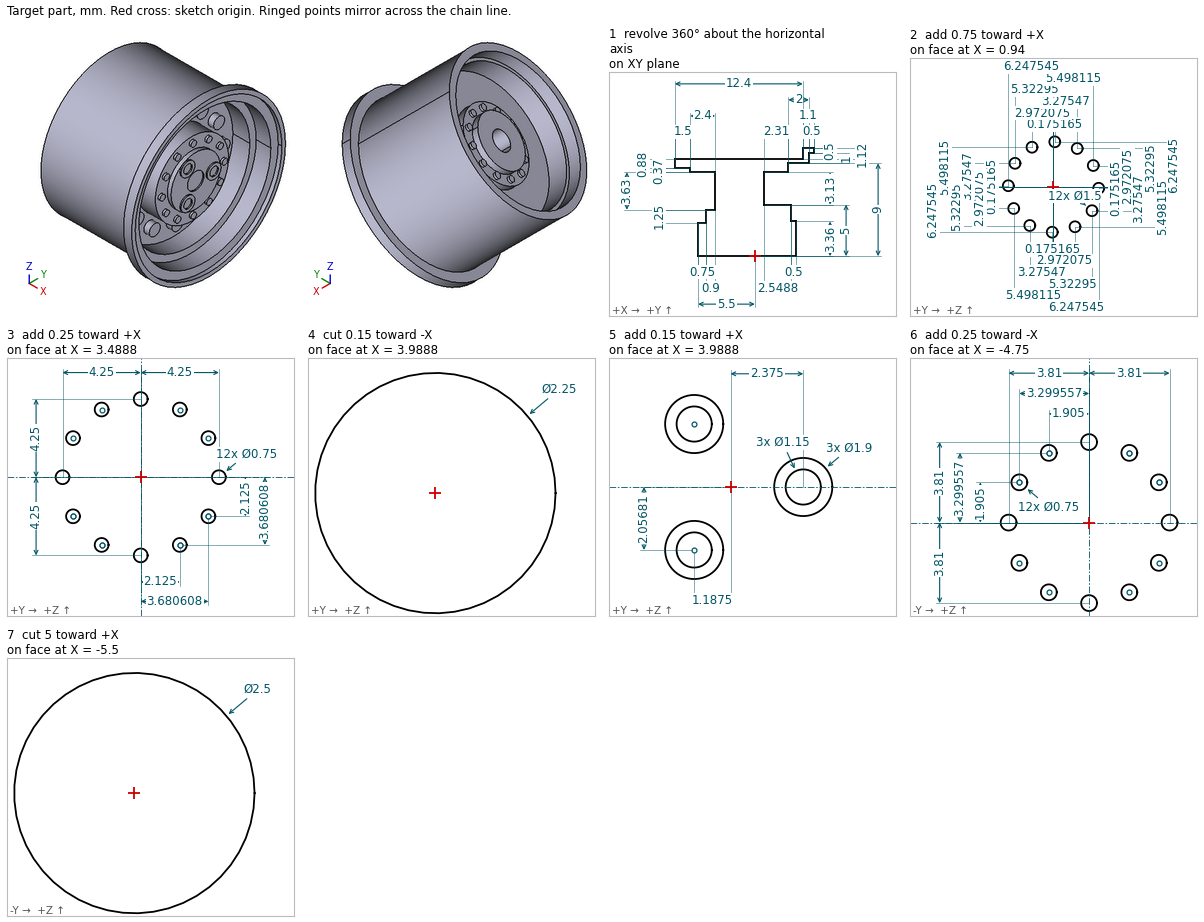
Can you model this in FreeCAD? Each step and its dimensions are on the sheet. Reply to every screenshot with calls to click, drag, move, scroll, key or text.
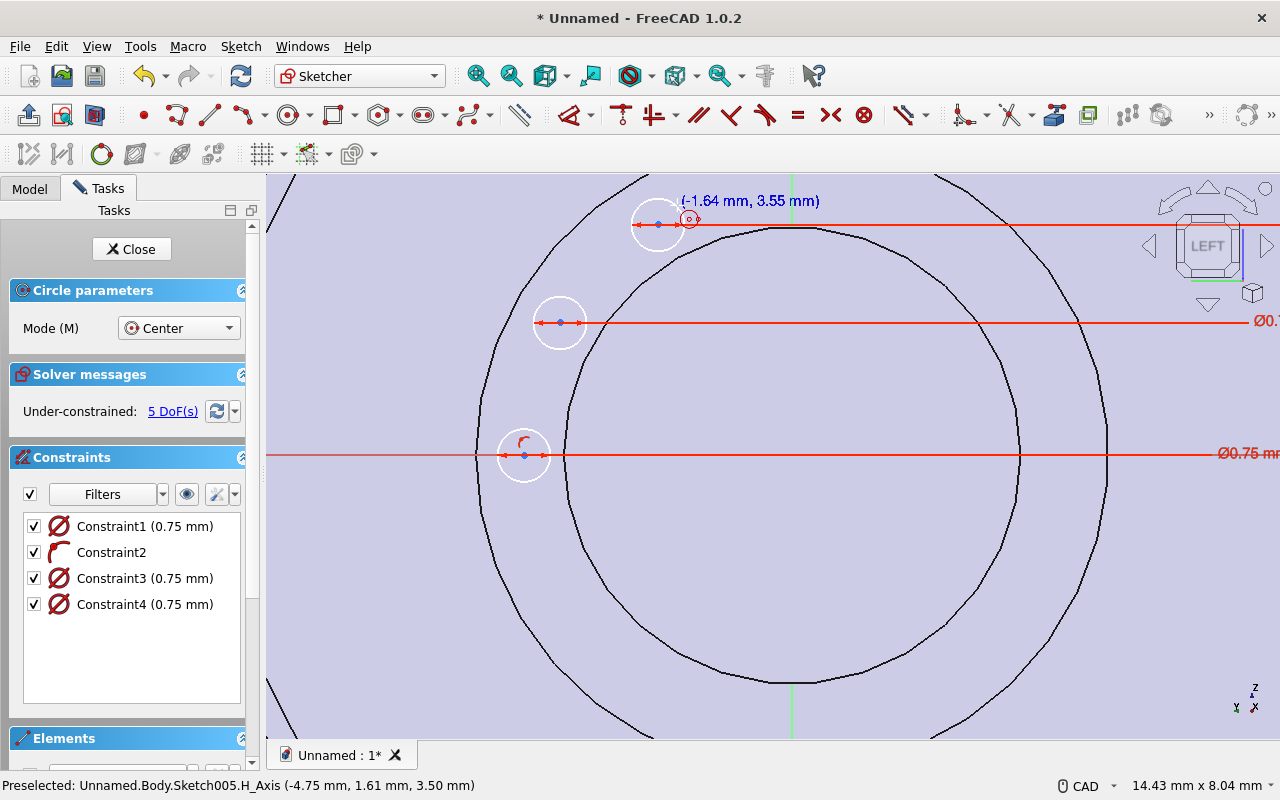
scroll(526, 459, down, 2)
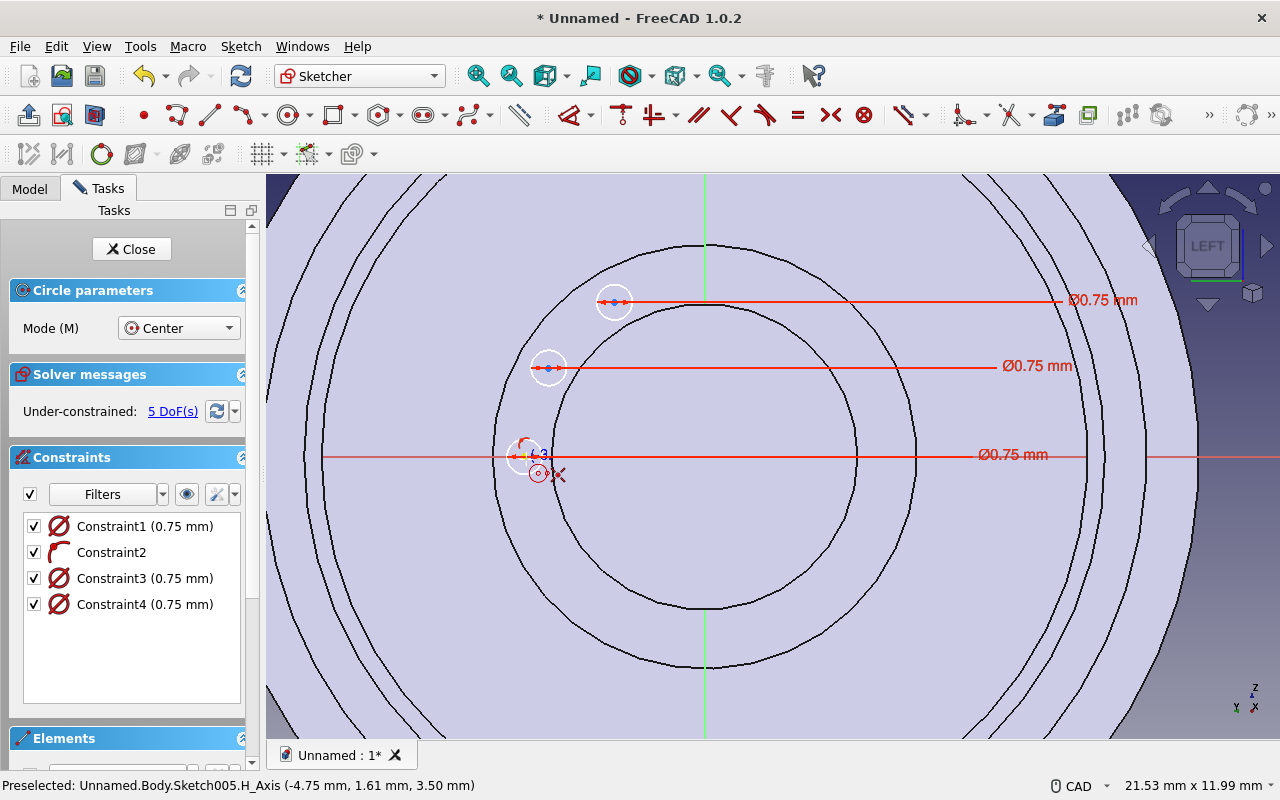
scroll(705, 277, up, 2)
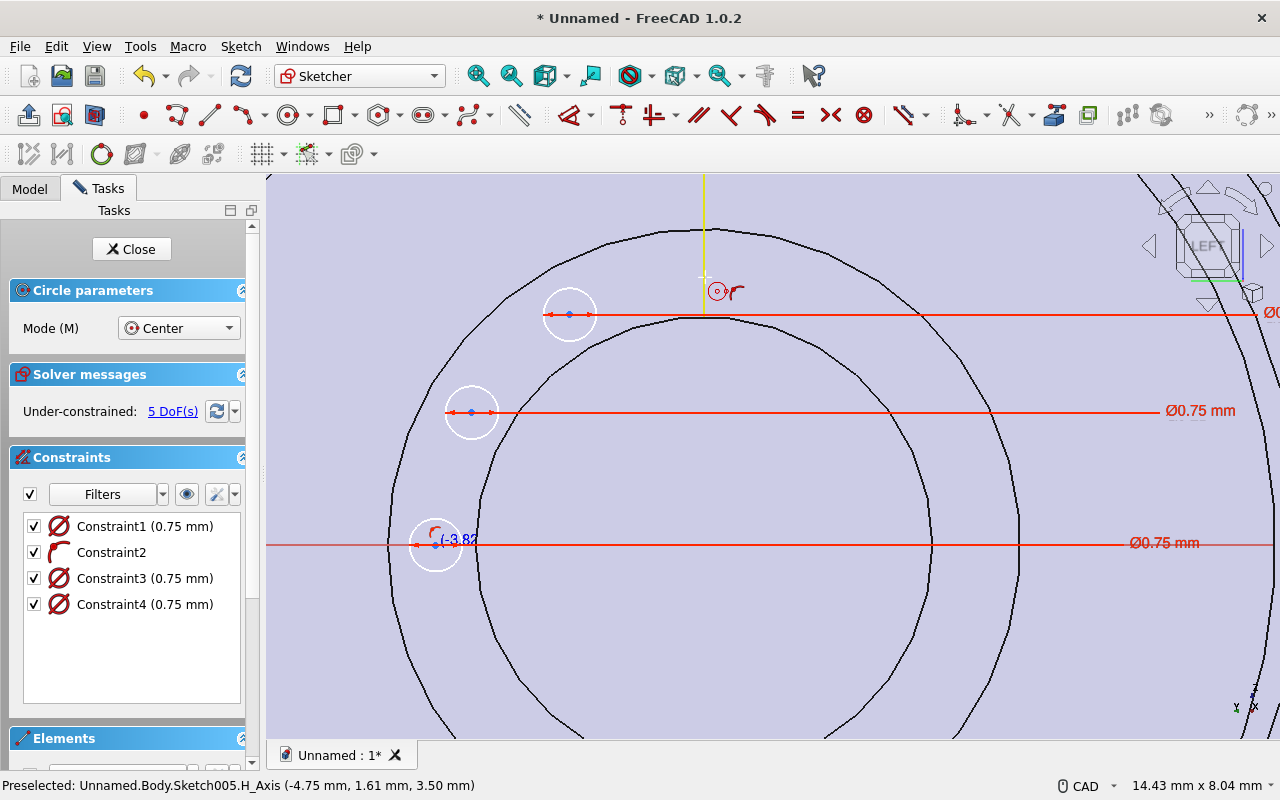
click(704, 277)
move(723, 259)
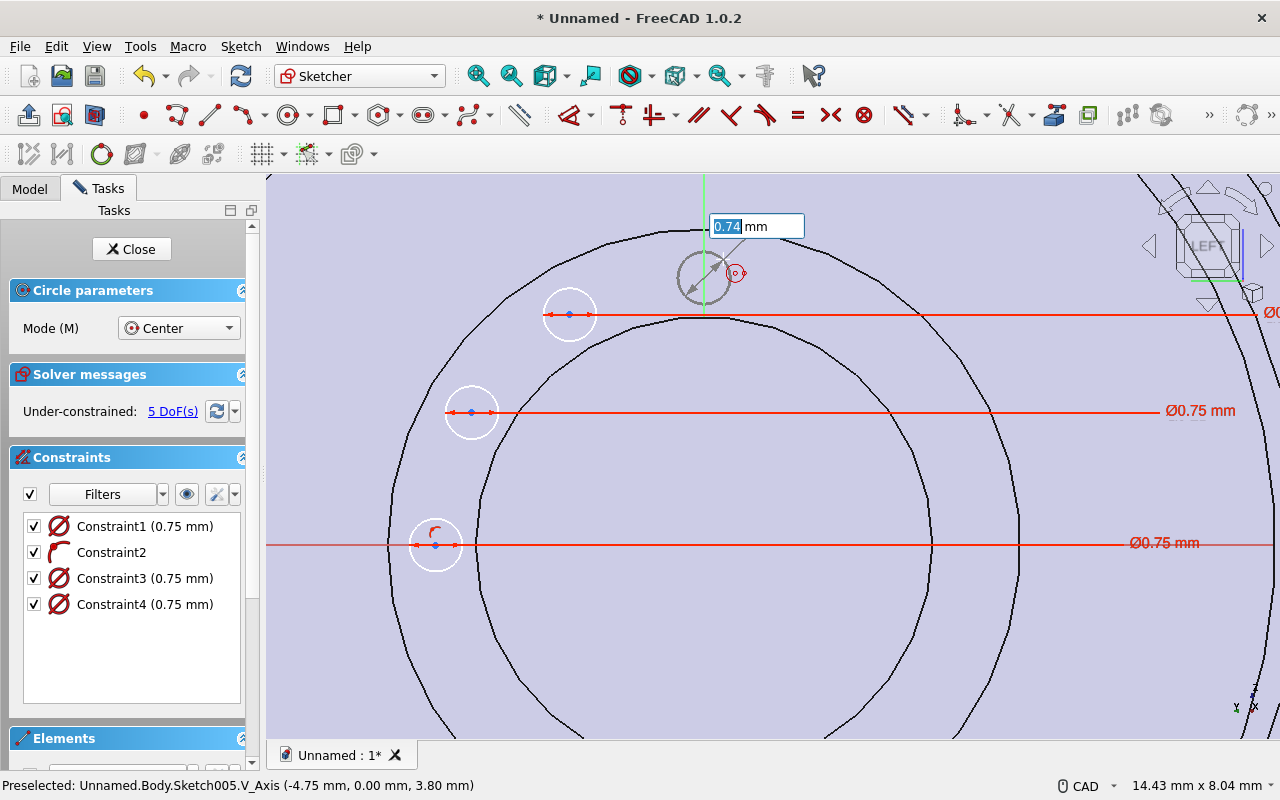
text(0.75)
key(Return)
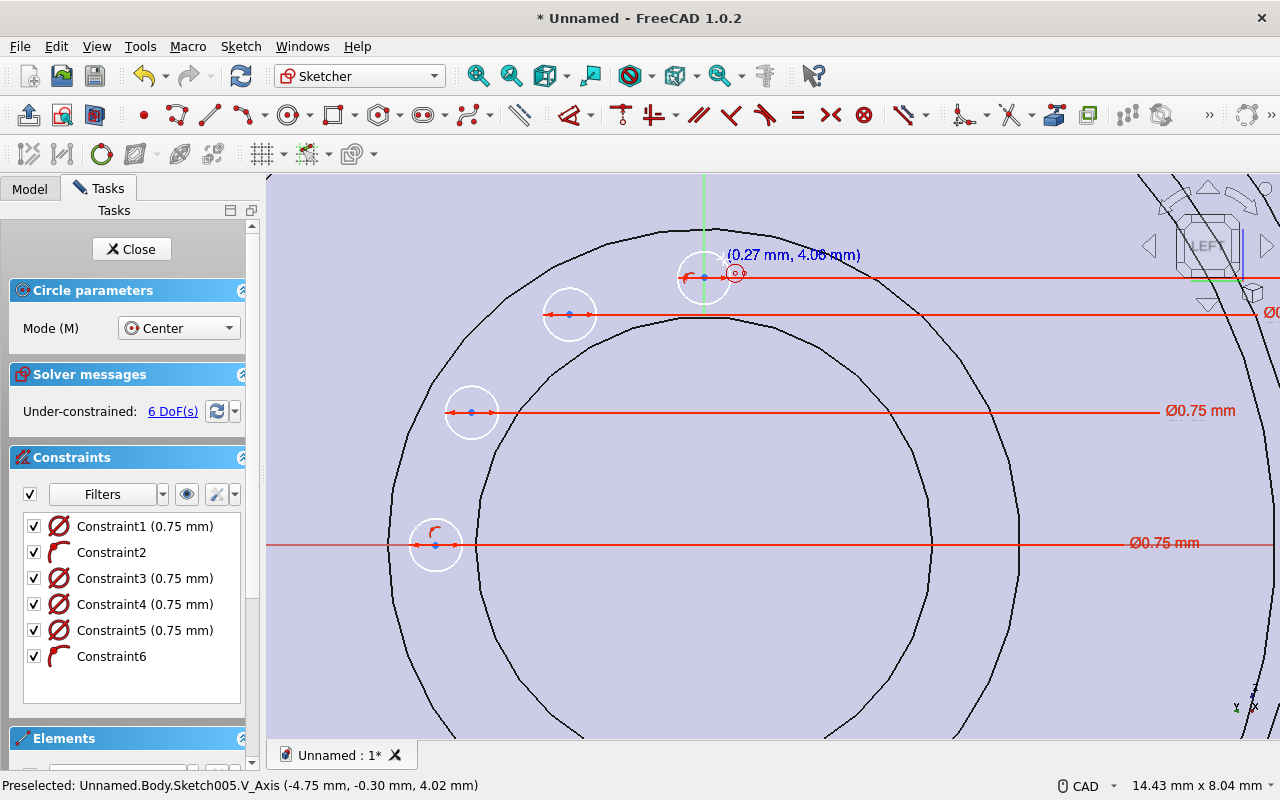
click(838, 313)
move(857, 295)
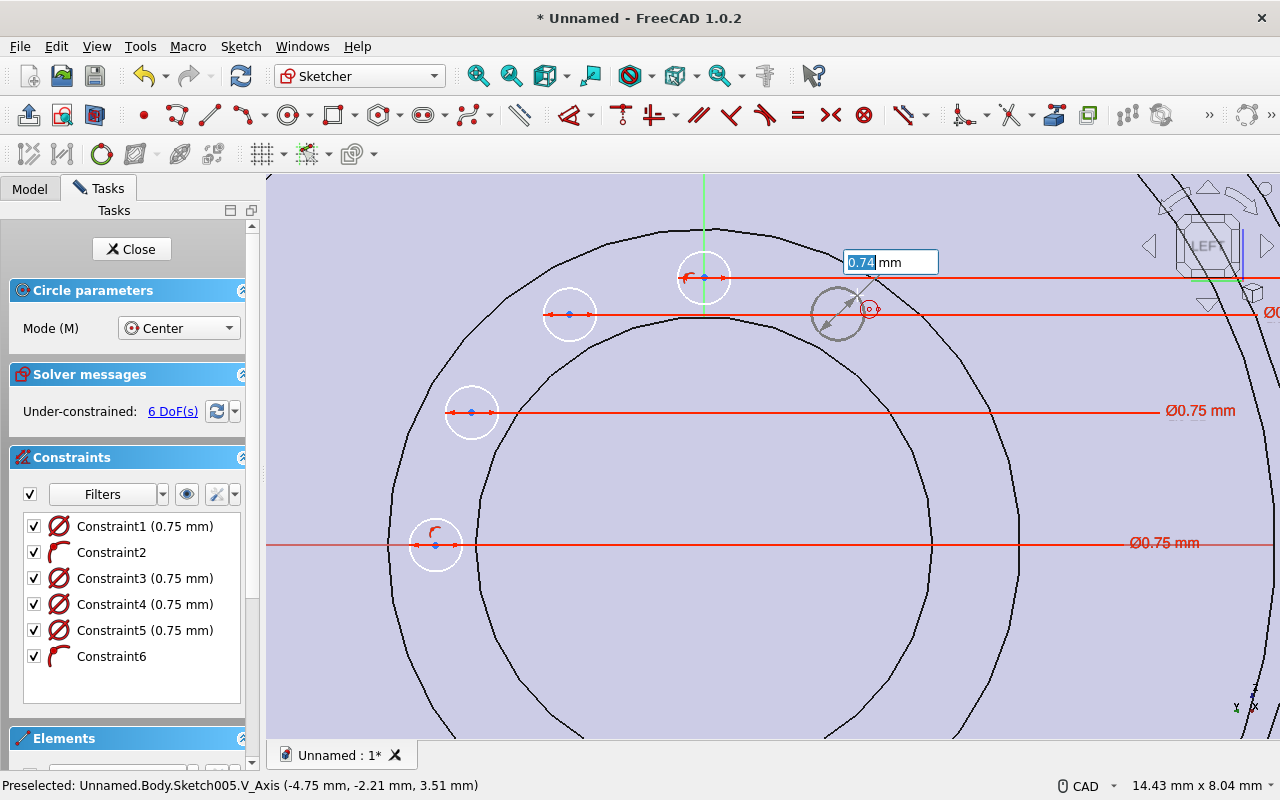
text(0.75)
key(Return)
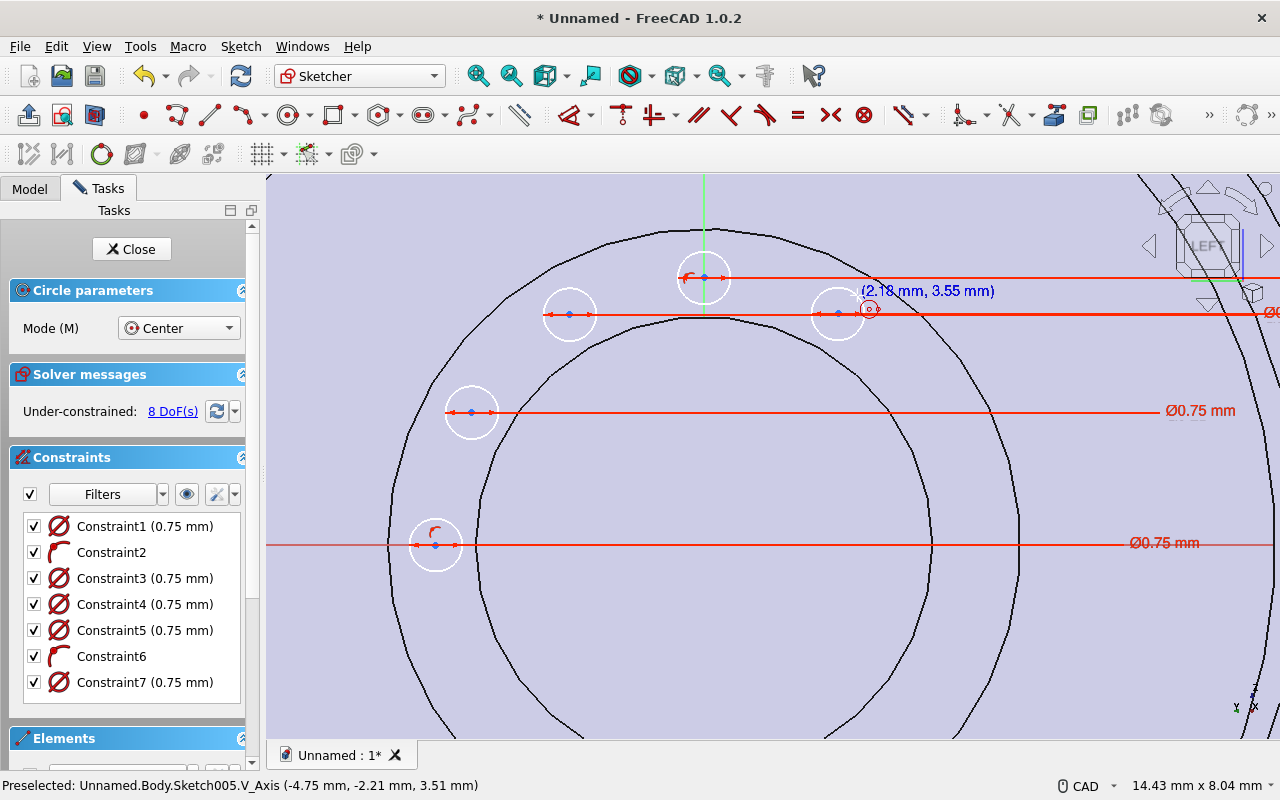
click(936, 411)
move(955, 393)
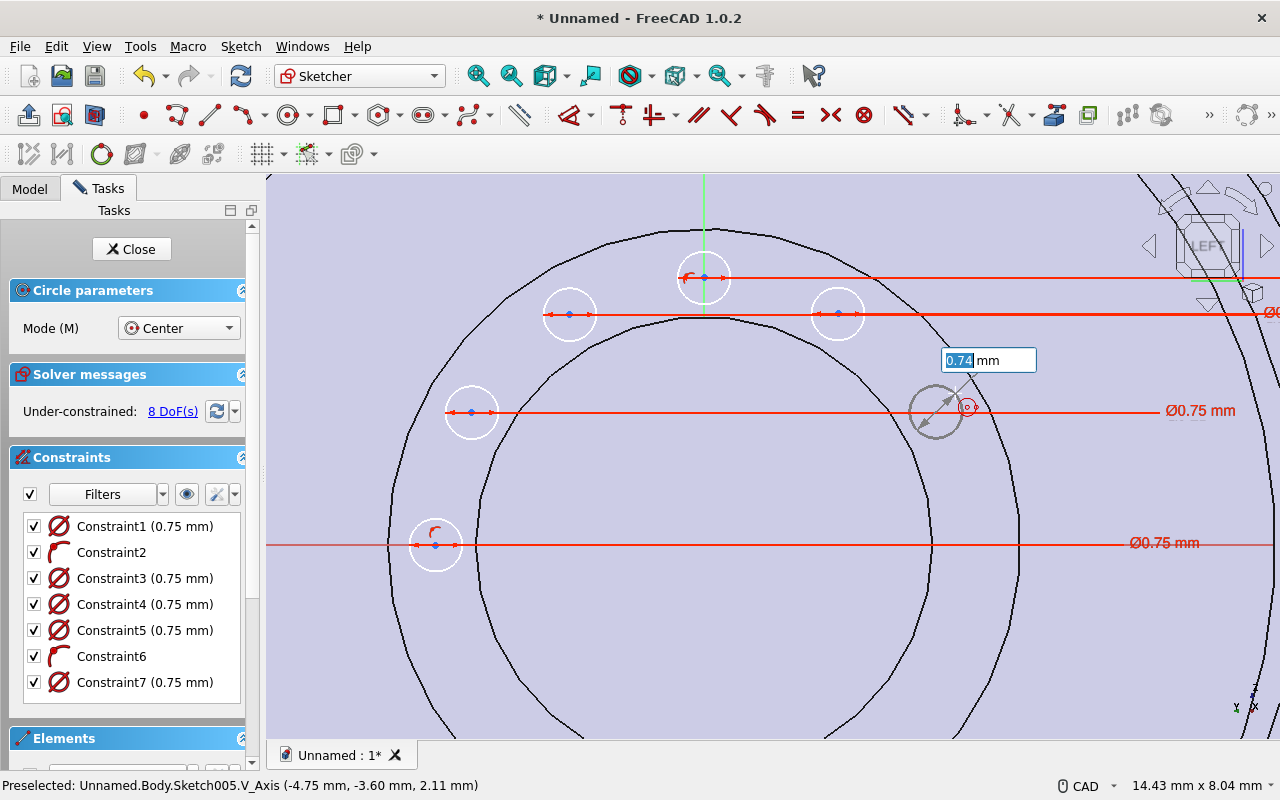
text(0.75)
key(Return)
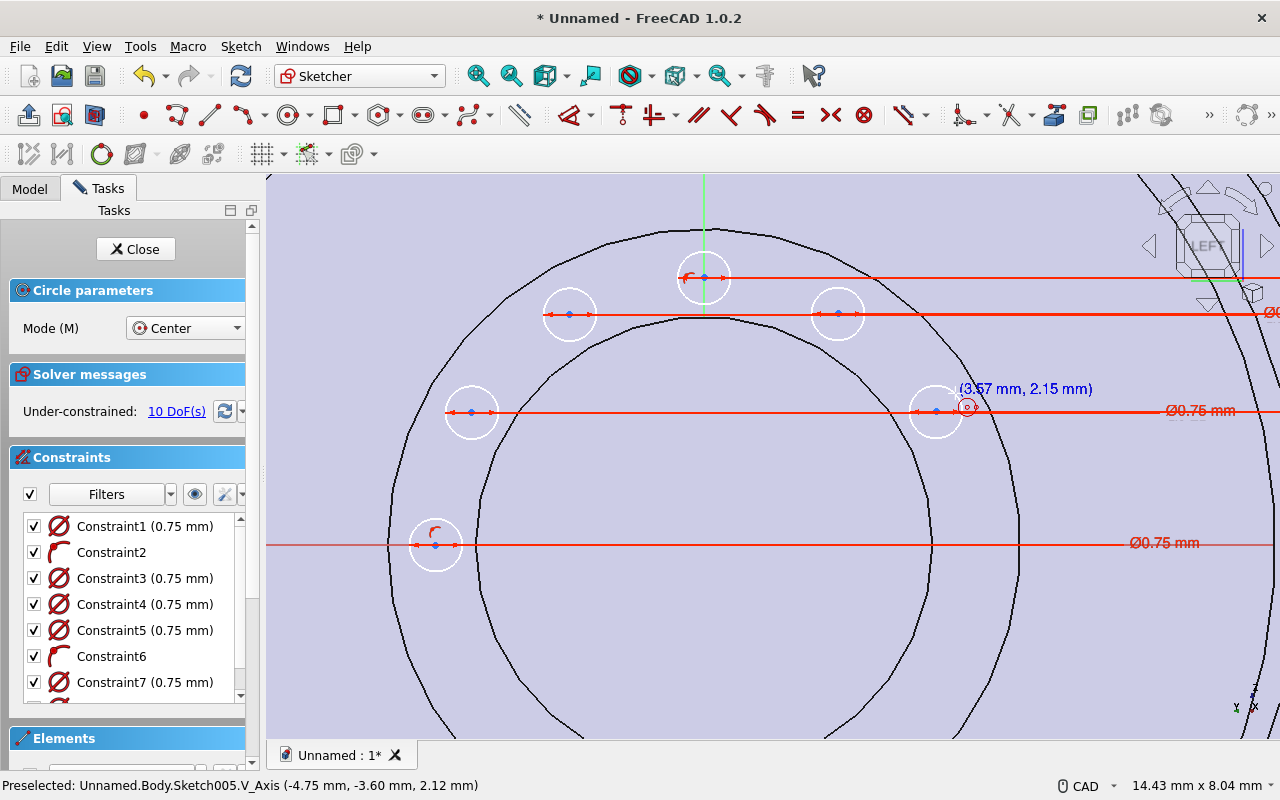
click(972, 545)
move(990, 527)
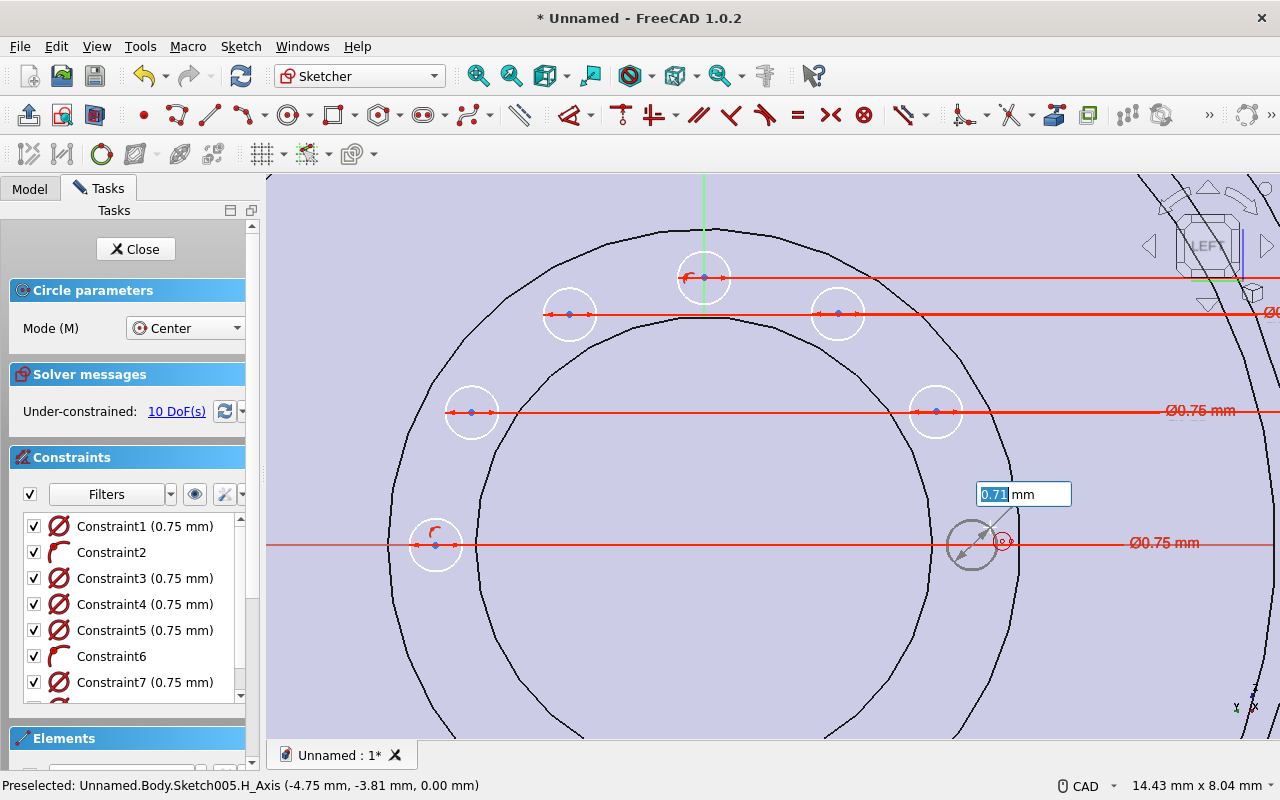
text(0.75)
key(Return)